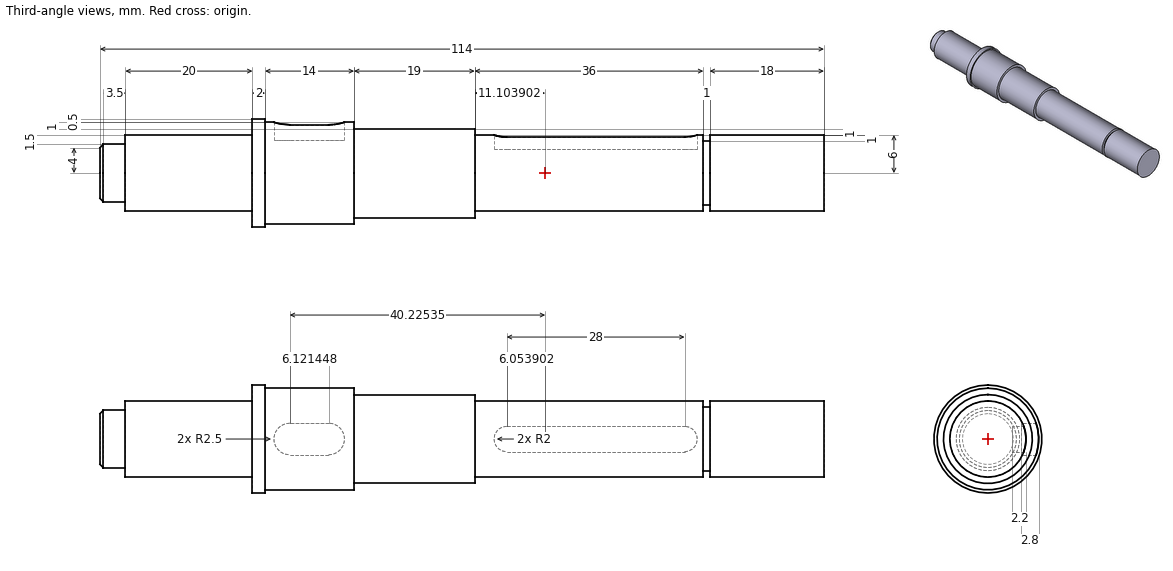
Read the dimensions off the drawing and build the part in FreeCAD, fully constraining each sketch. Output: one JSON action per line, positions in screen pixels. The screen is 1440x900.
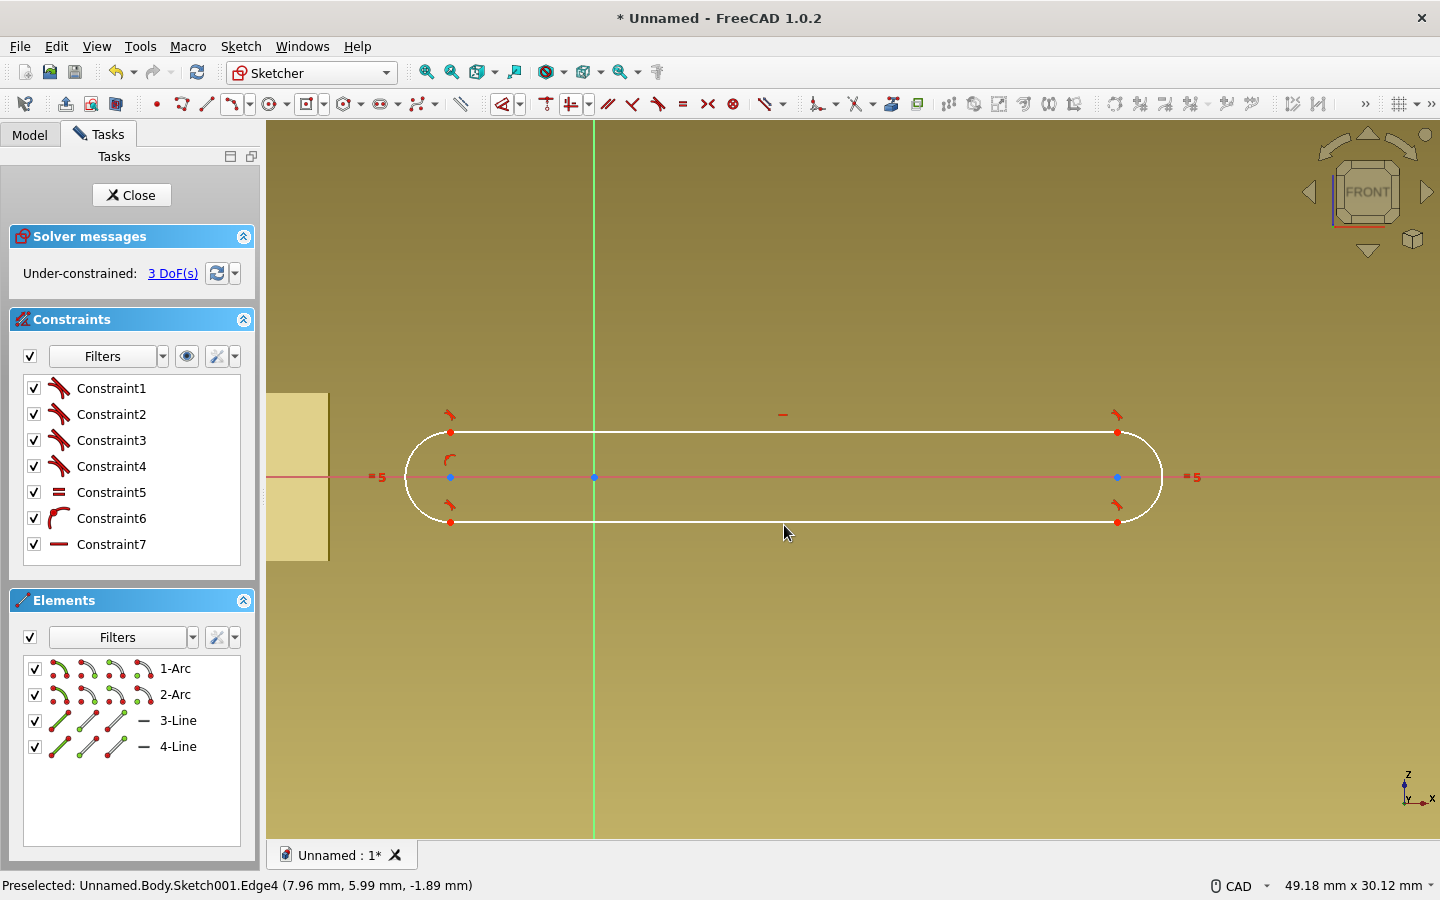
{"action": "left_click", "coordinate": [414, 451]}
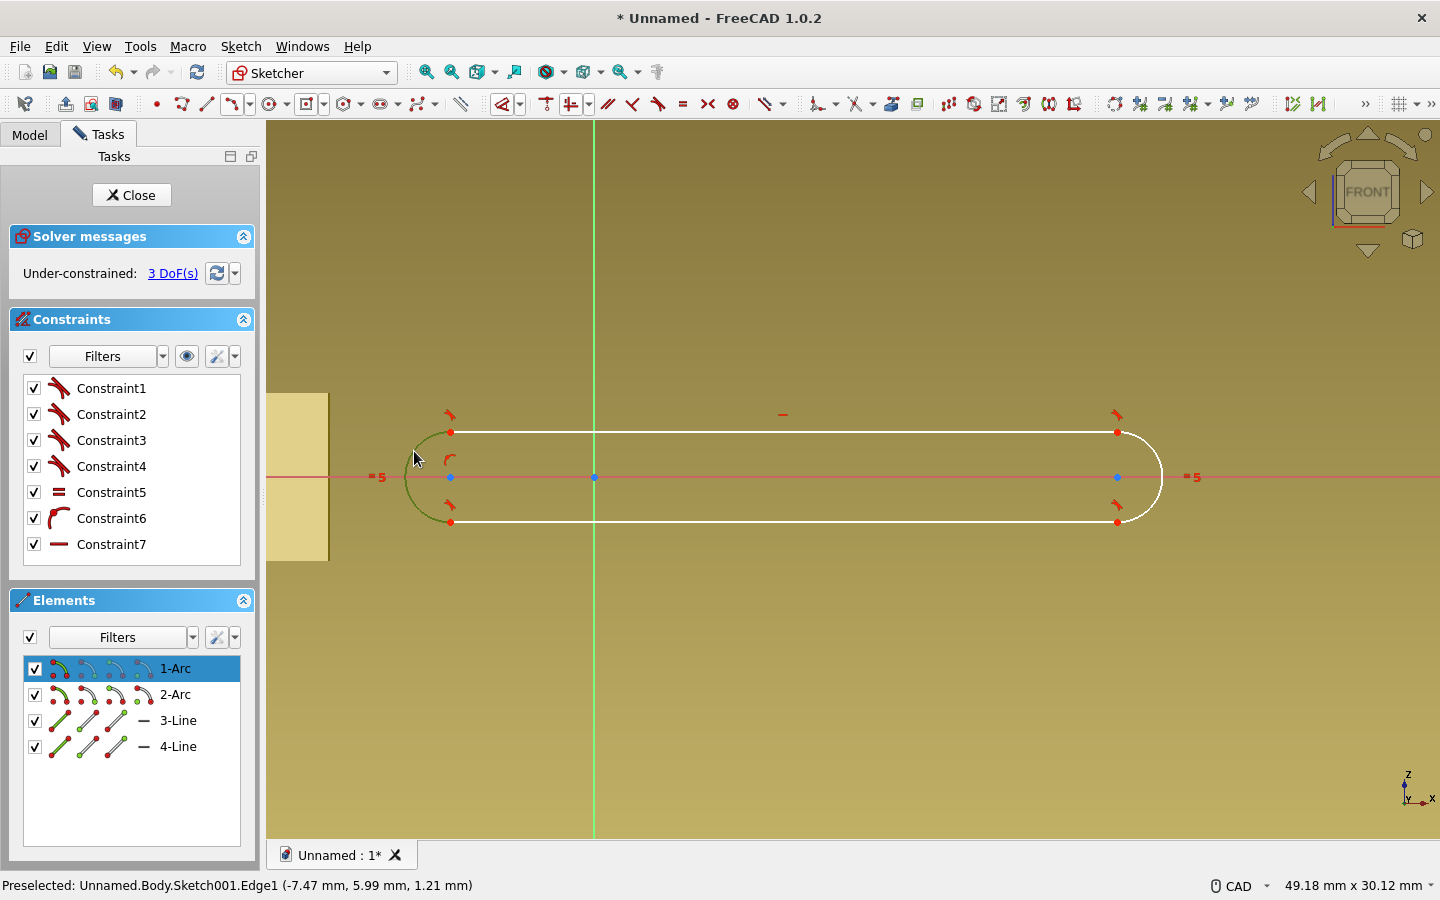
{"action": "key", "text": "k r"}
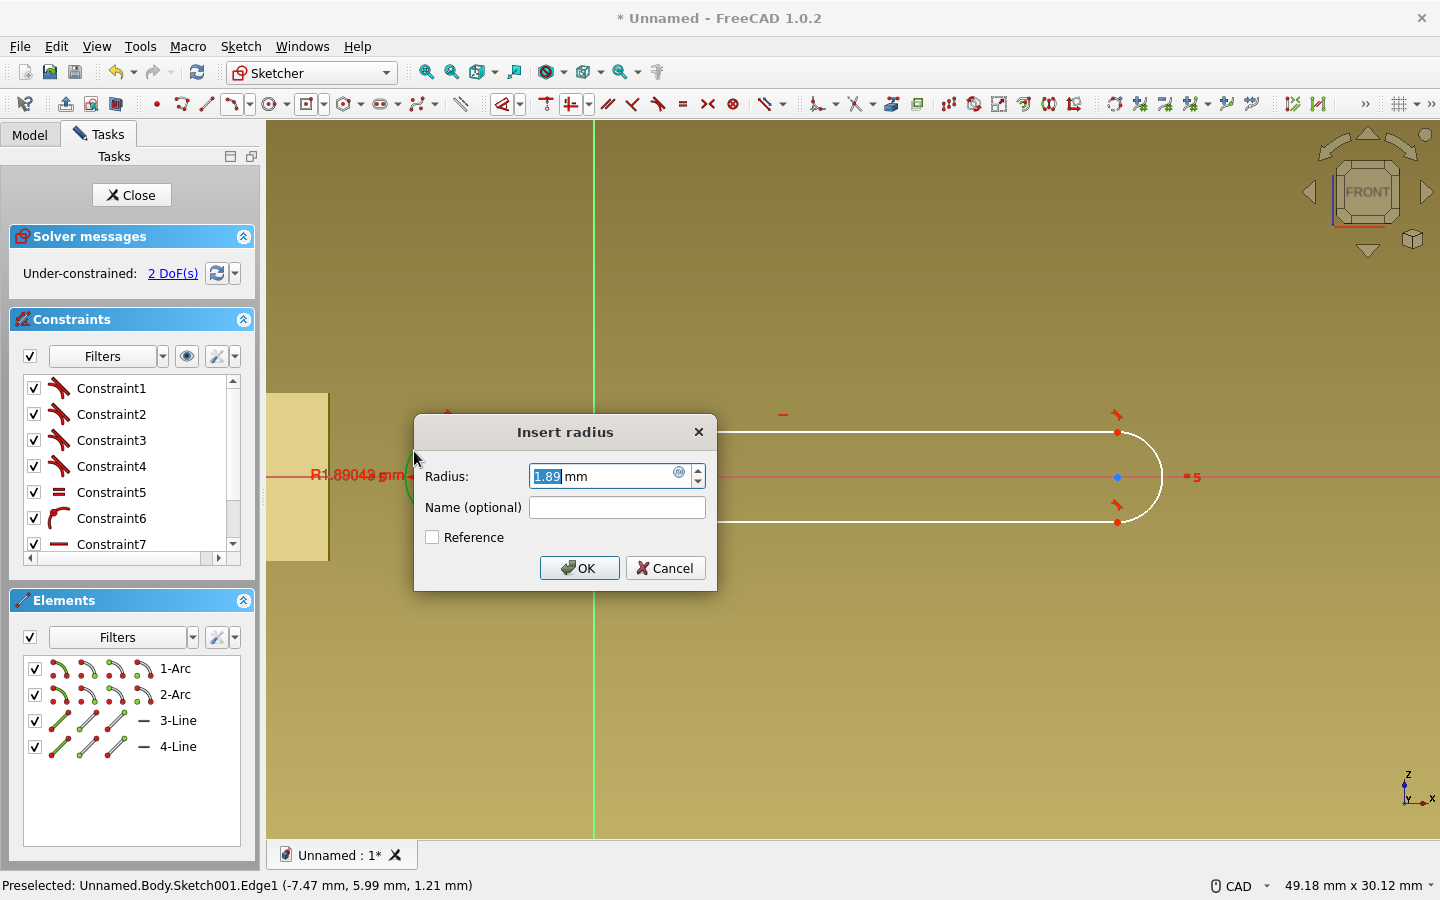
{"action": "type", "text": "2"}
{"action": "key", "text": "Return"}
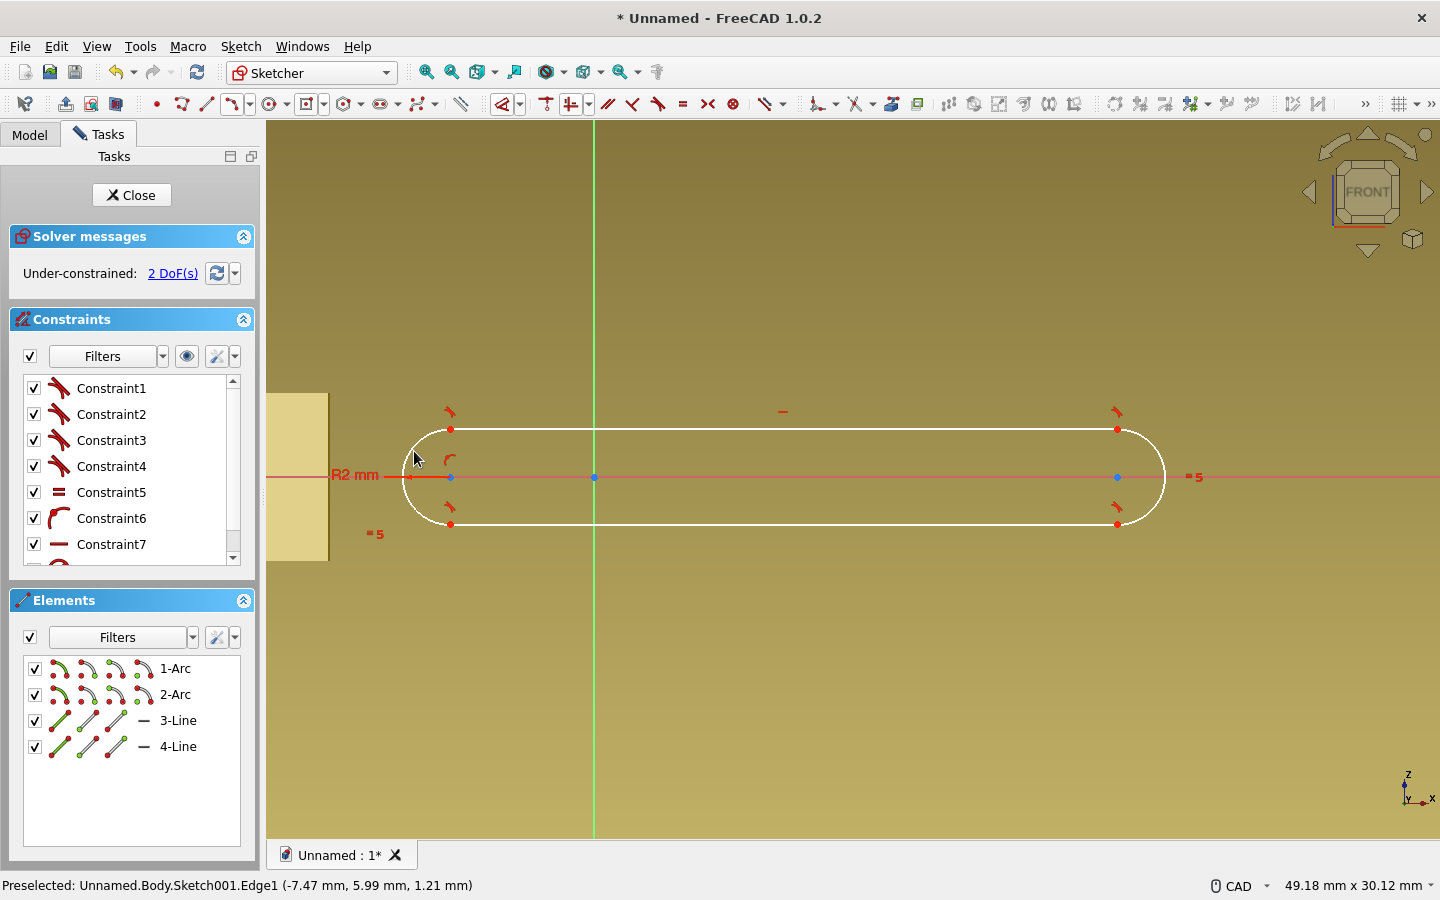
{"action": "left_click", "coordinate": [651, 429]}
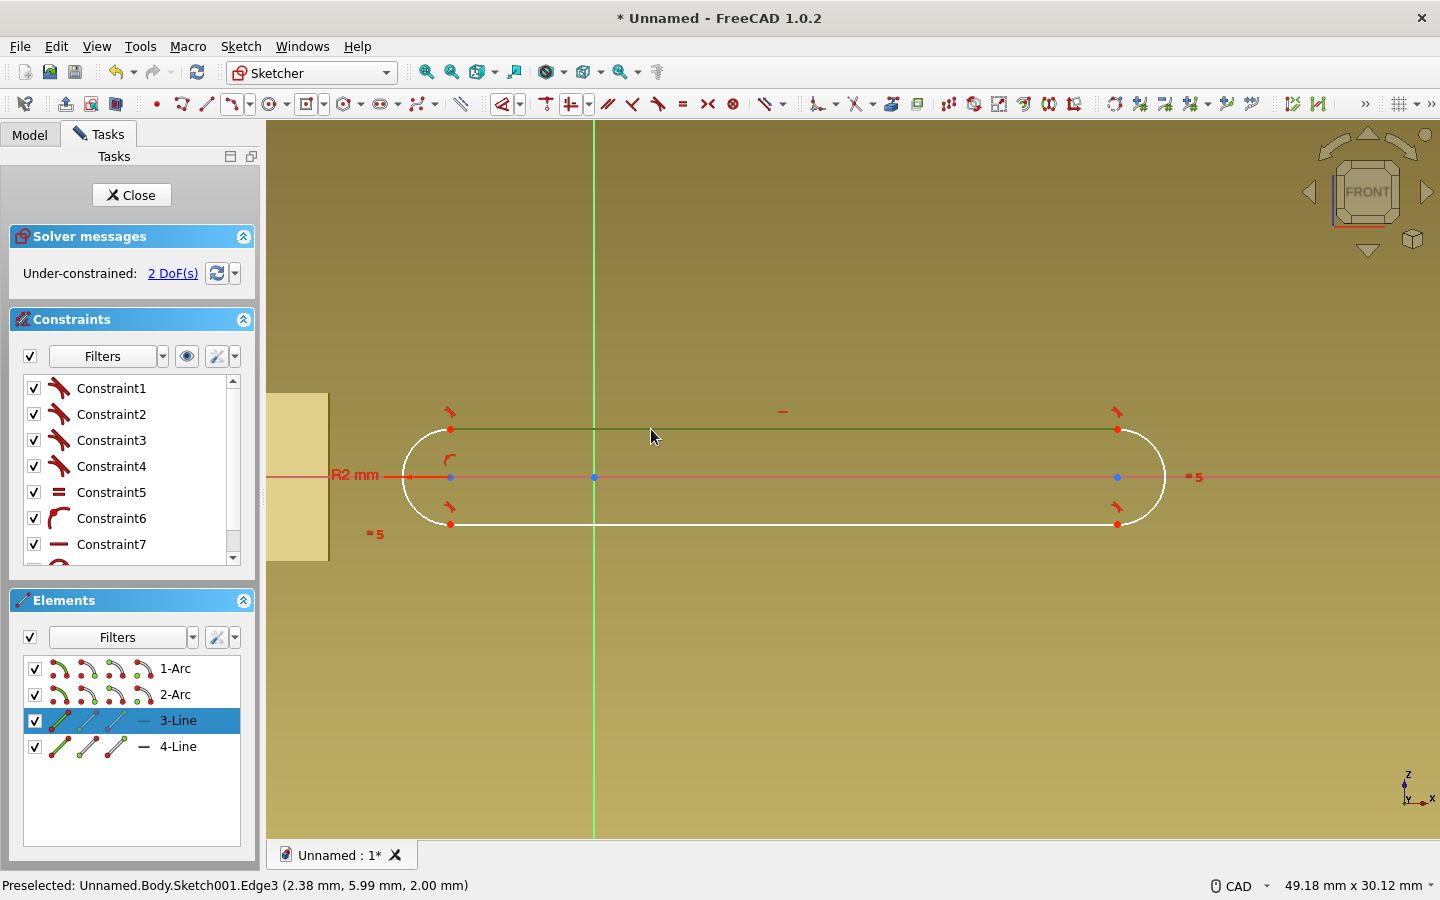
{"action": "left_click", "coordinate": [520, 104]}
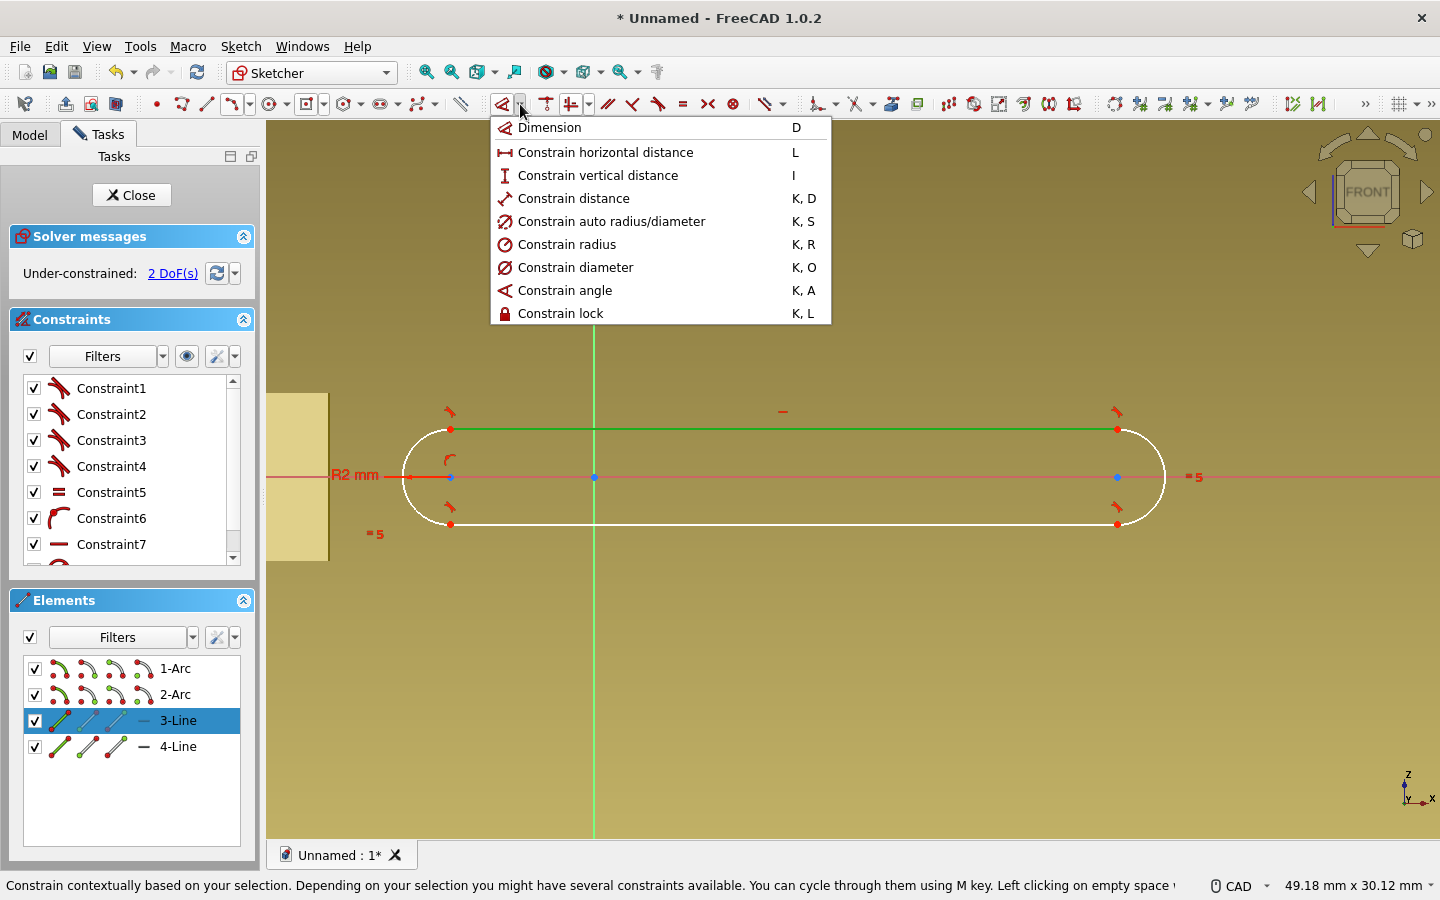
{"action": "left_click", "coordinate": [661, 152]}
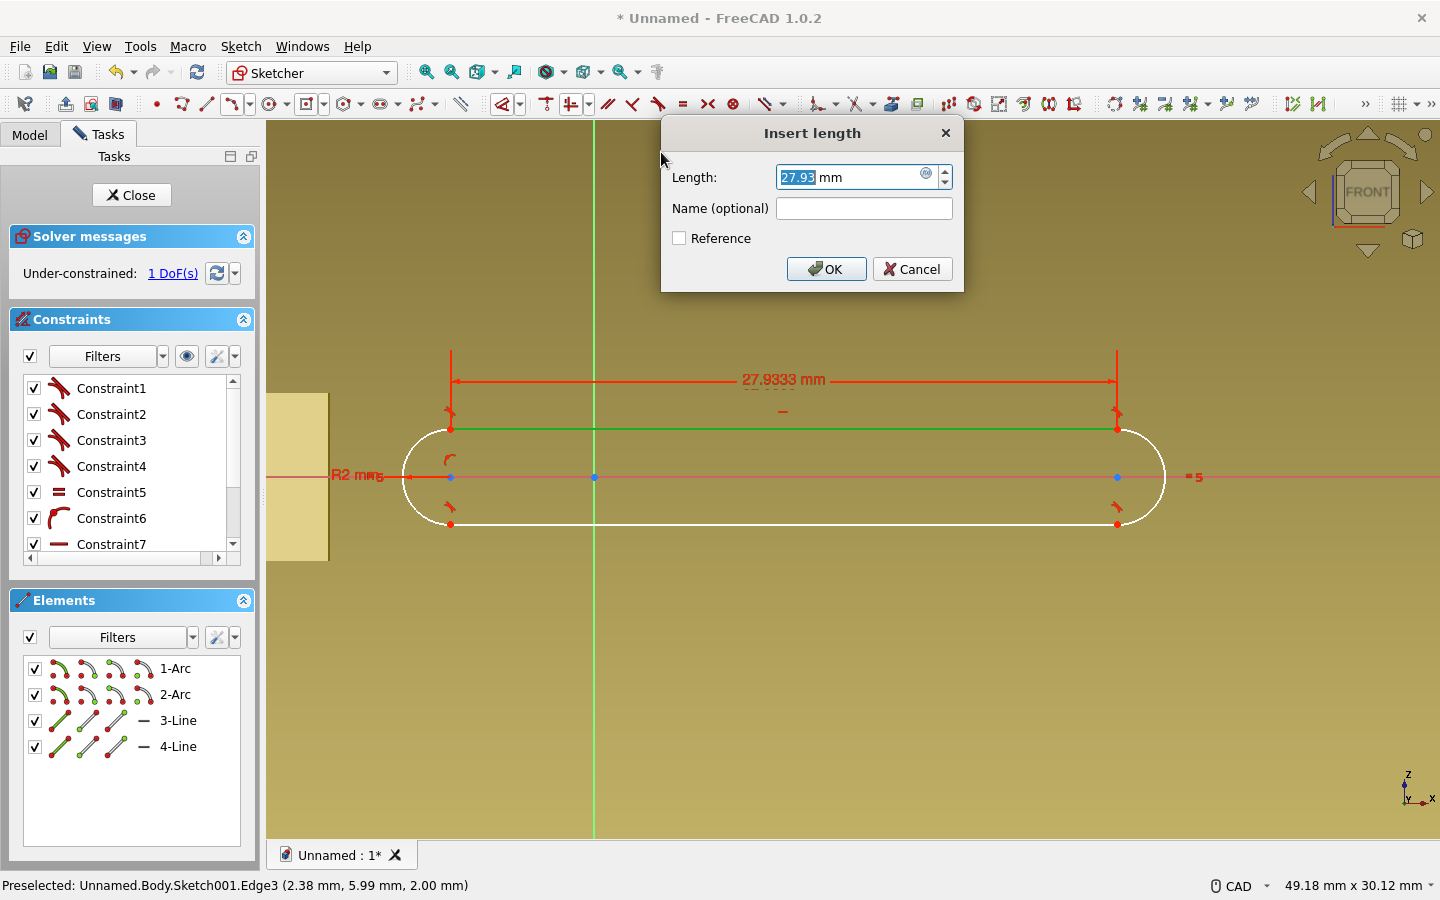
{"action": "type", "text": "28"}
{"action": "key", "text": "Return"}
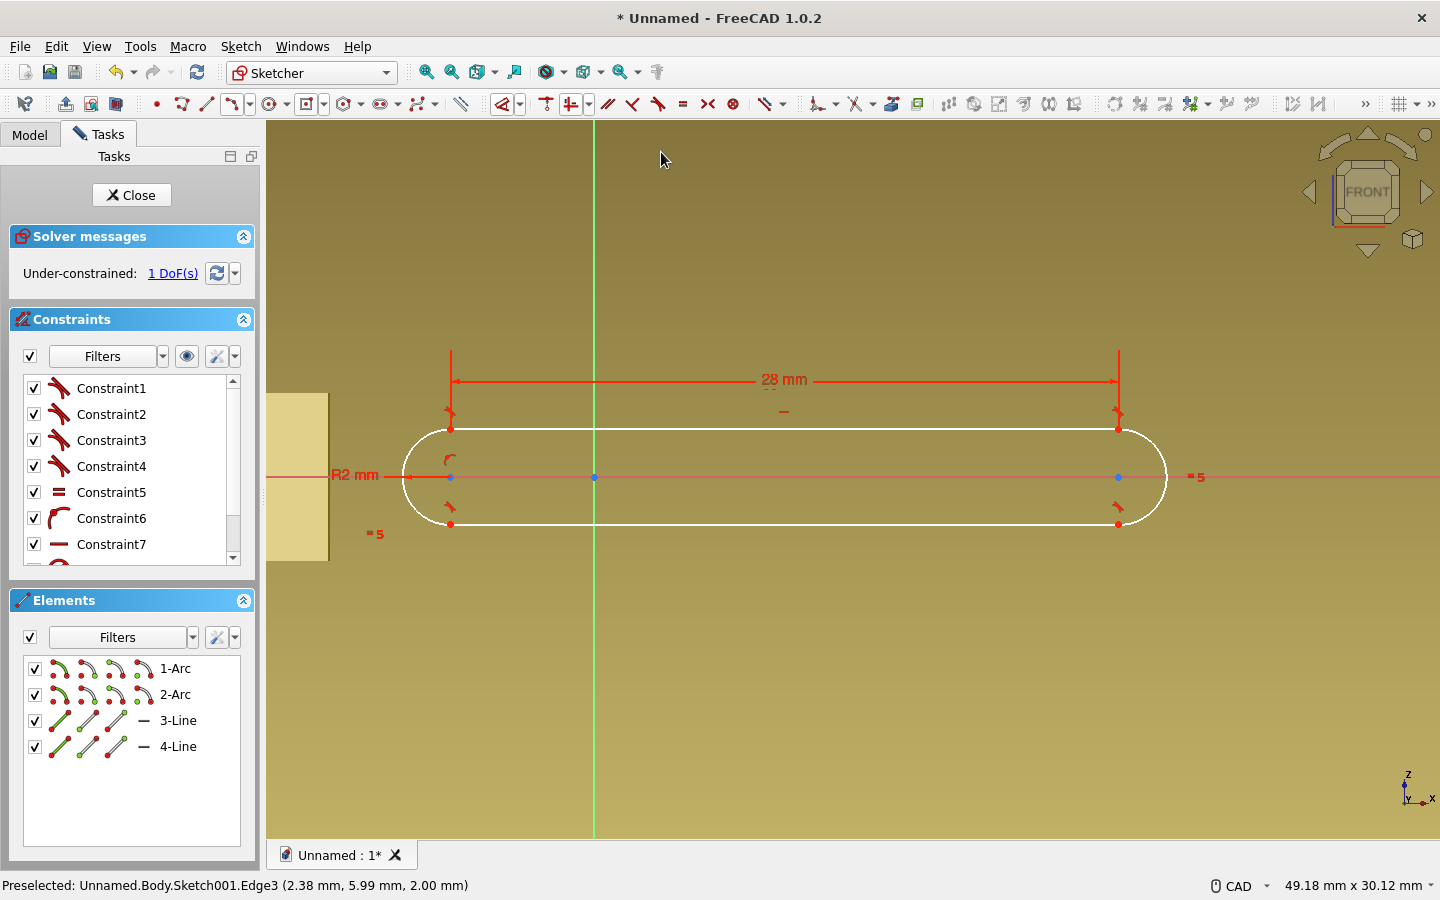
{"action": "left_click", "coordinate": [451, 429]}